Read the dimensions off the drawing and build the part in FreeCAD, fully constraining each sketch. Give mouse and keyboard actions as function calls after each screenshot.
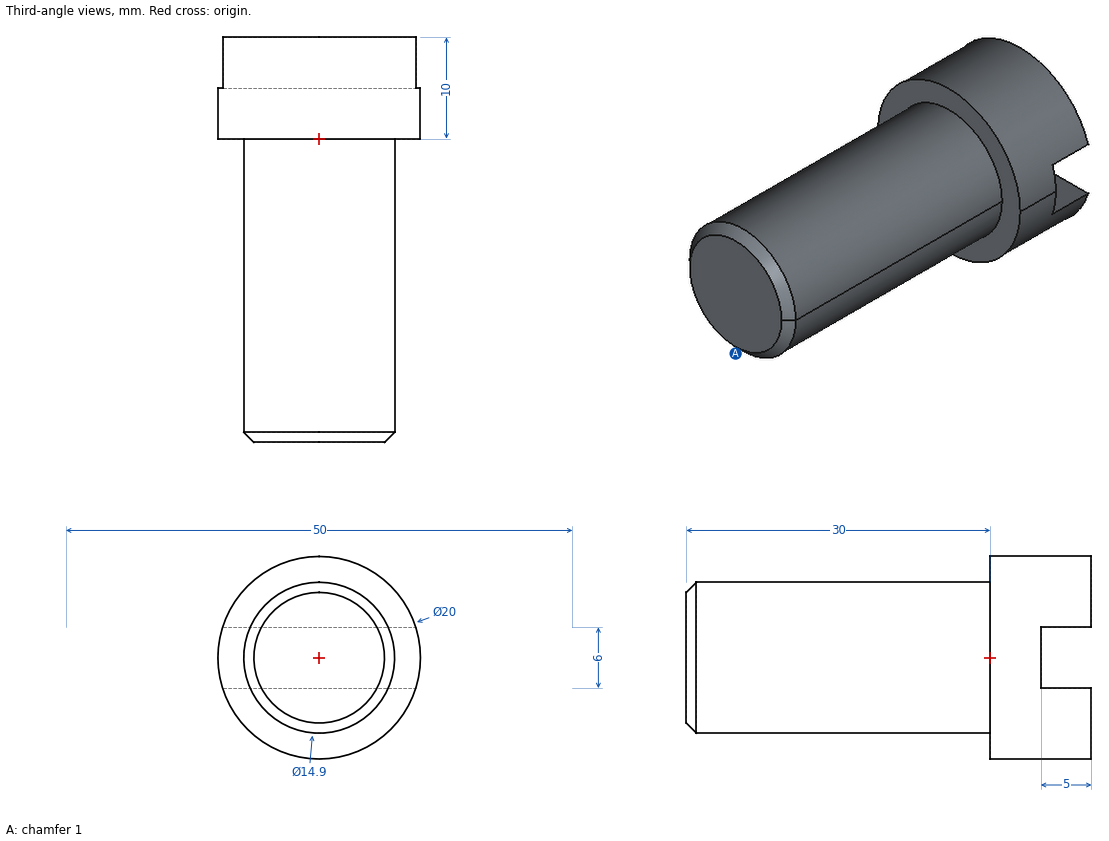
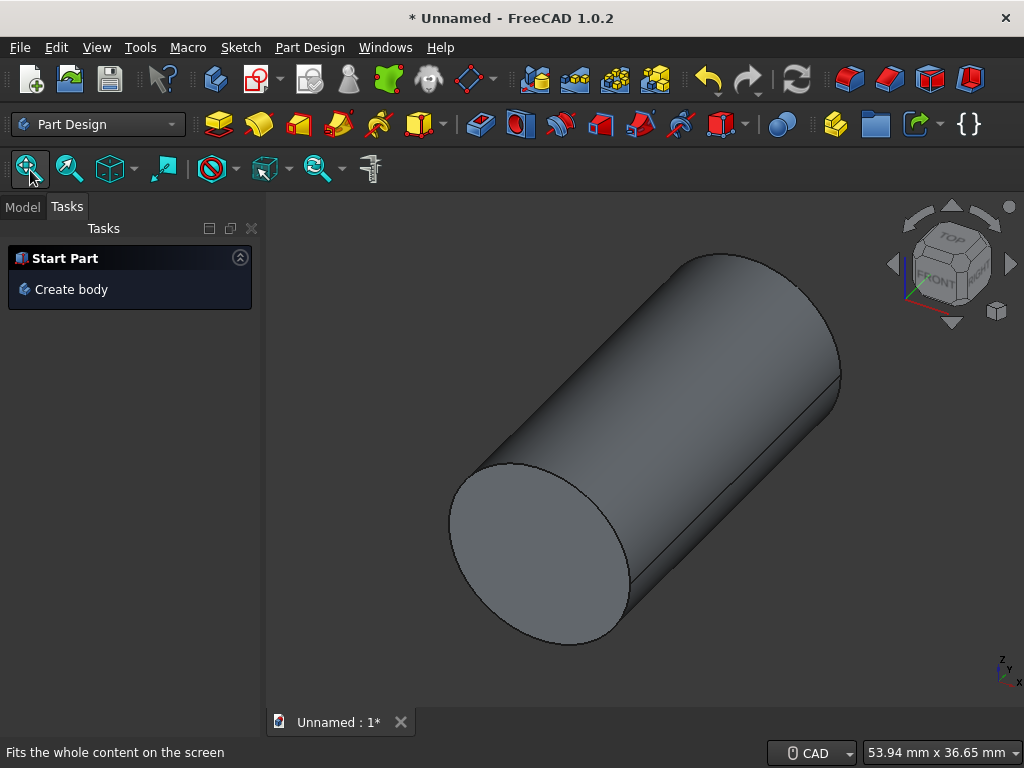
click(256, 80)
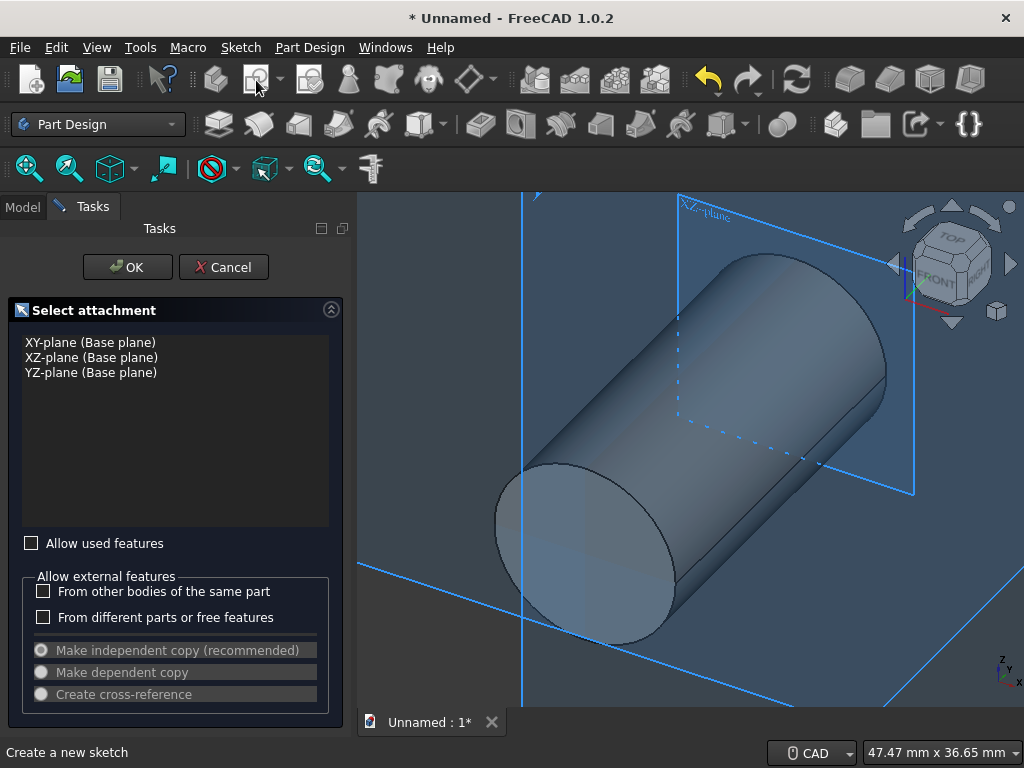
click(82, 358)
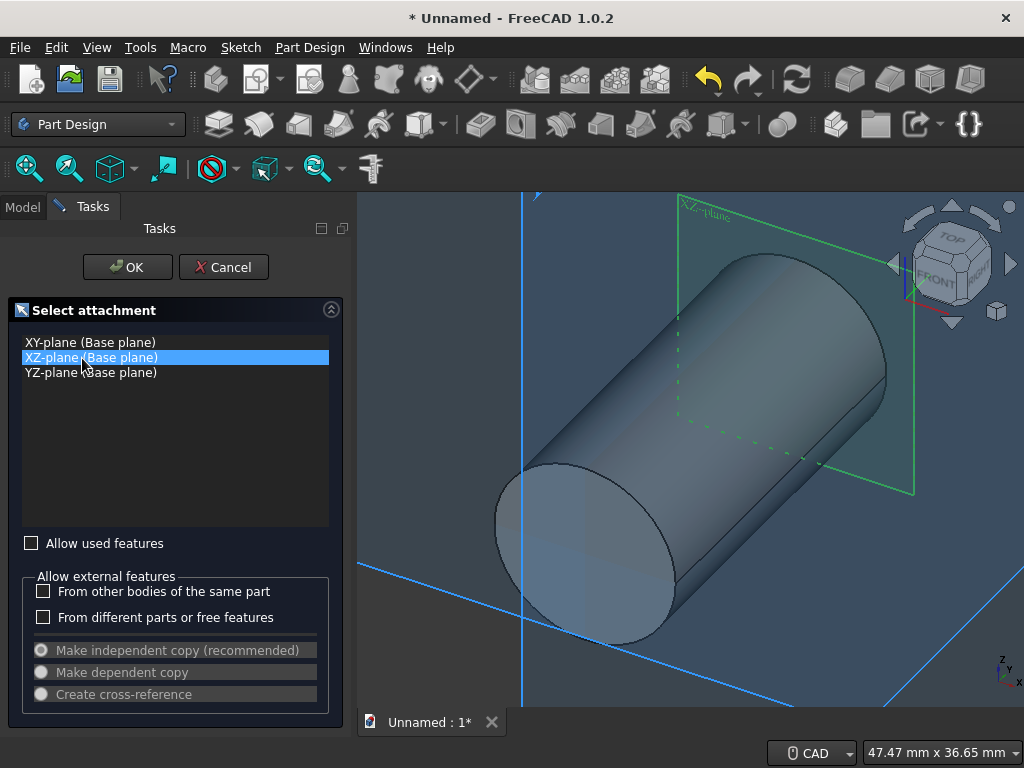
click(128, 267)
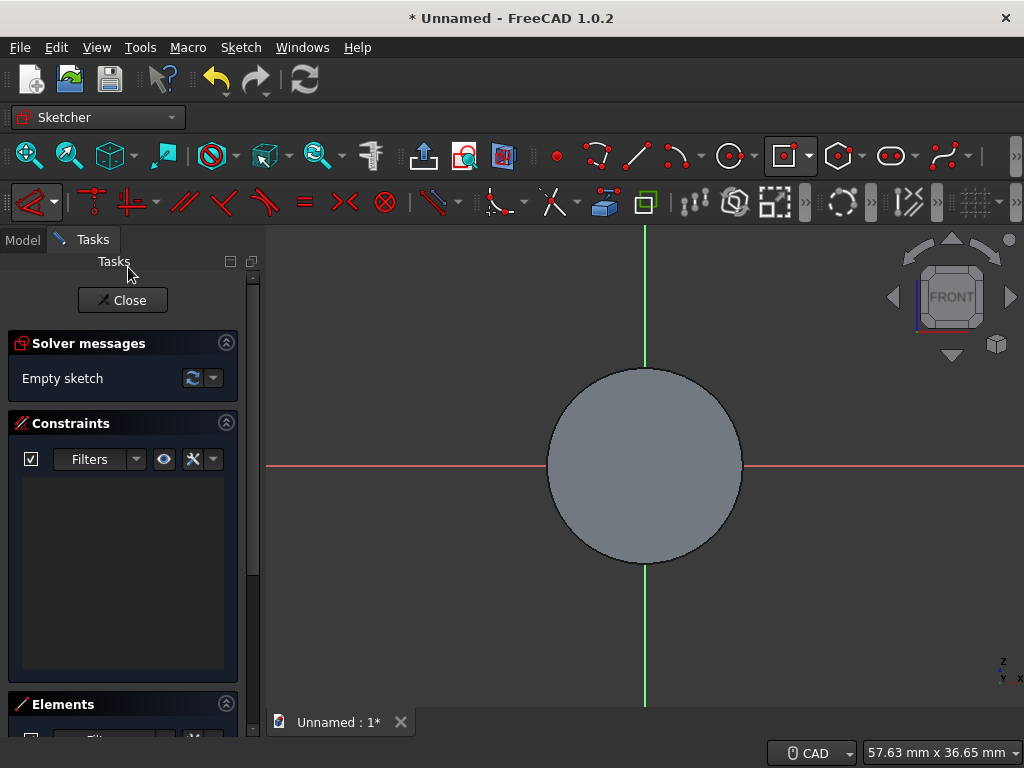
click(504, 156)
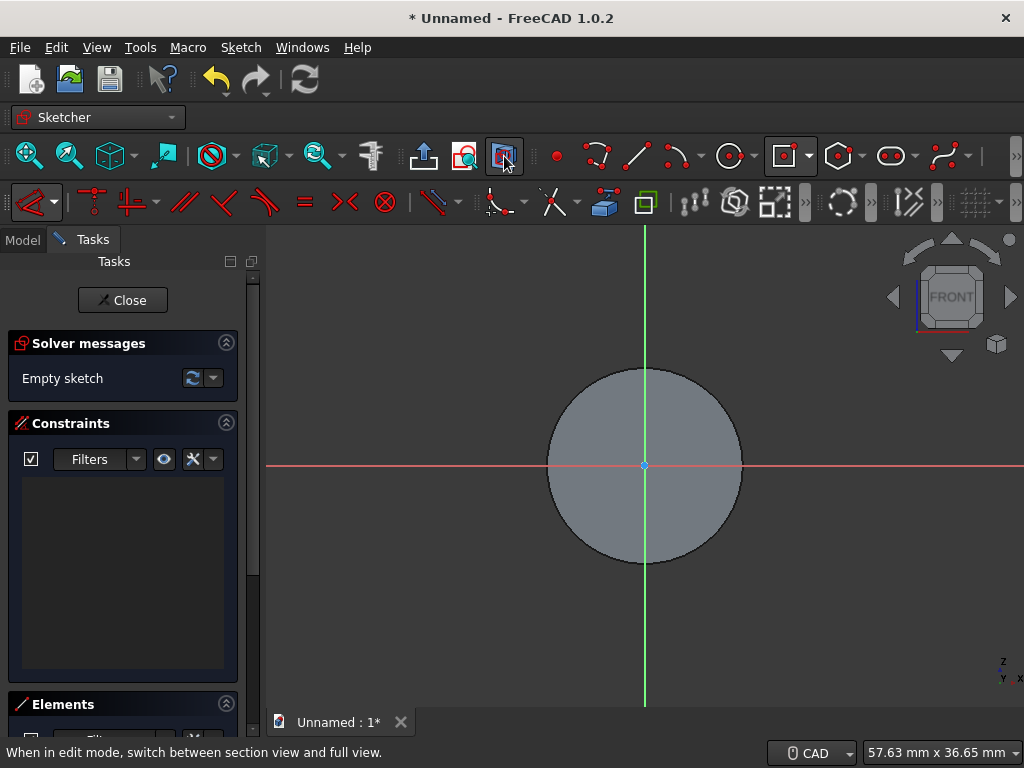
click(730, 156)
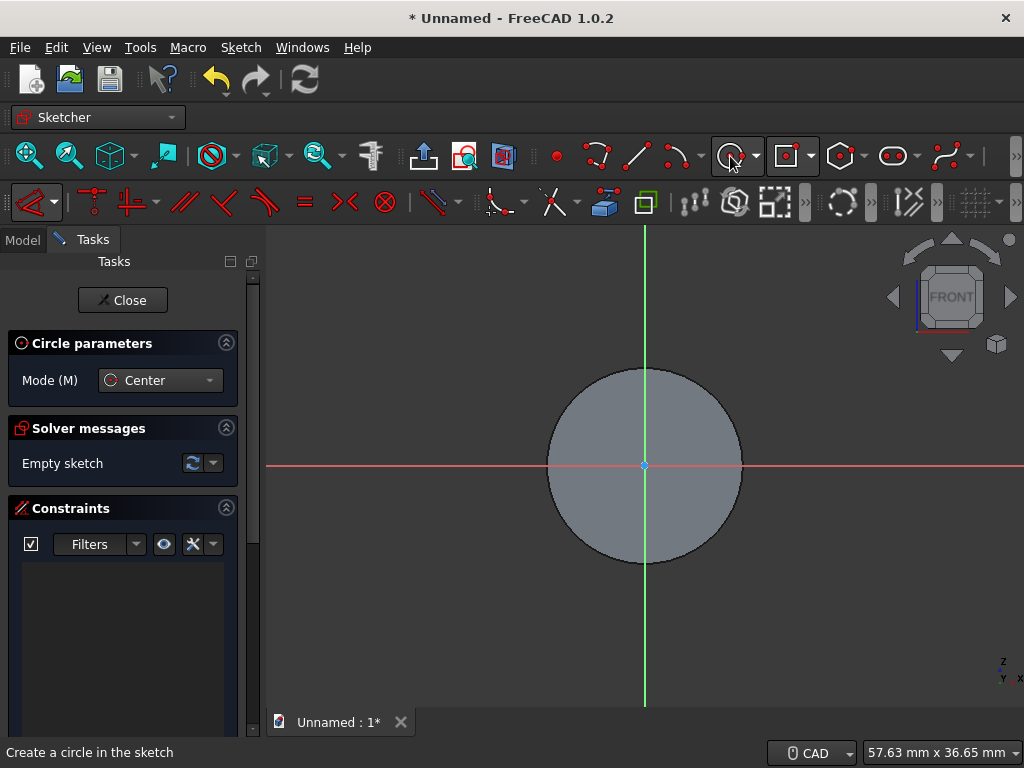
click(645, 466)
move(738, 373)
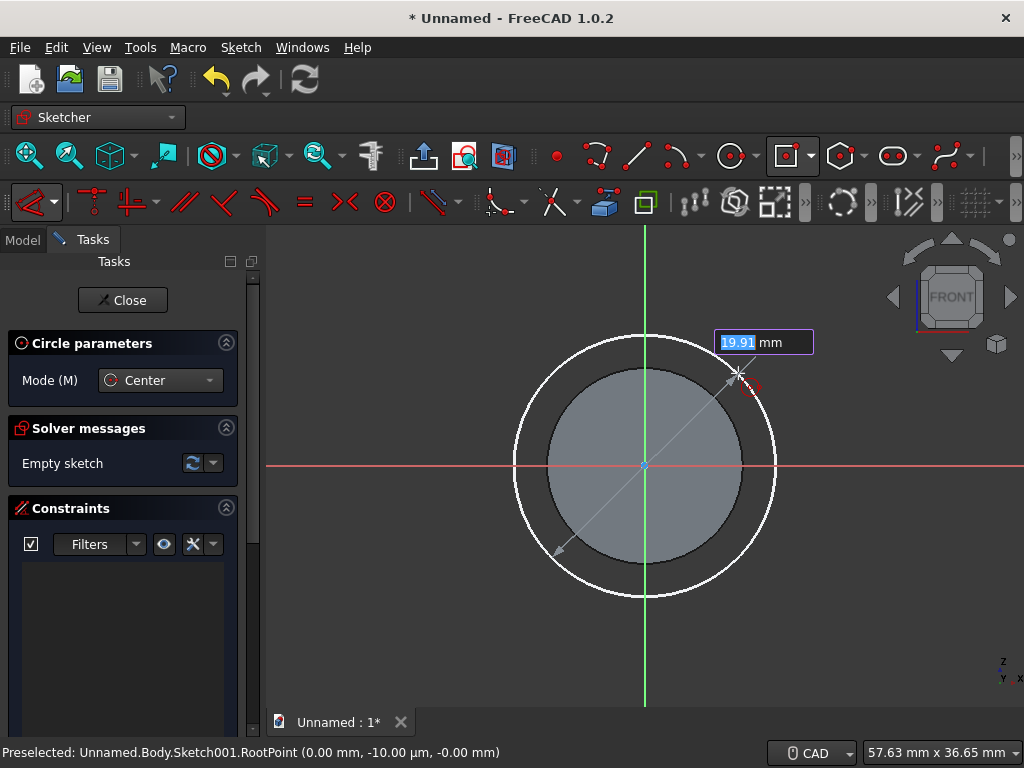
text(20)
key(Return)
key(Escape)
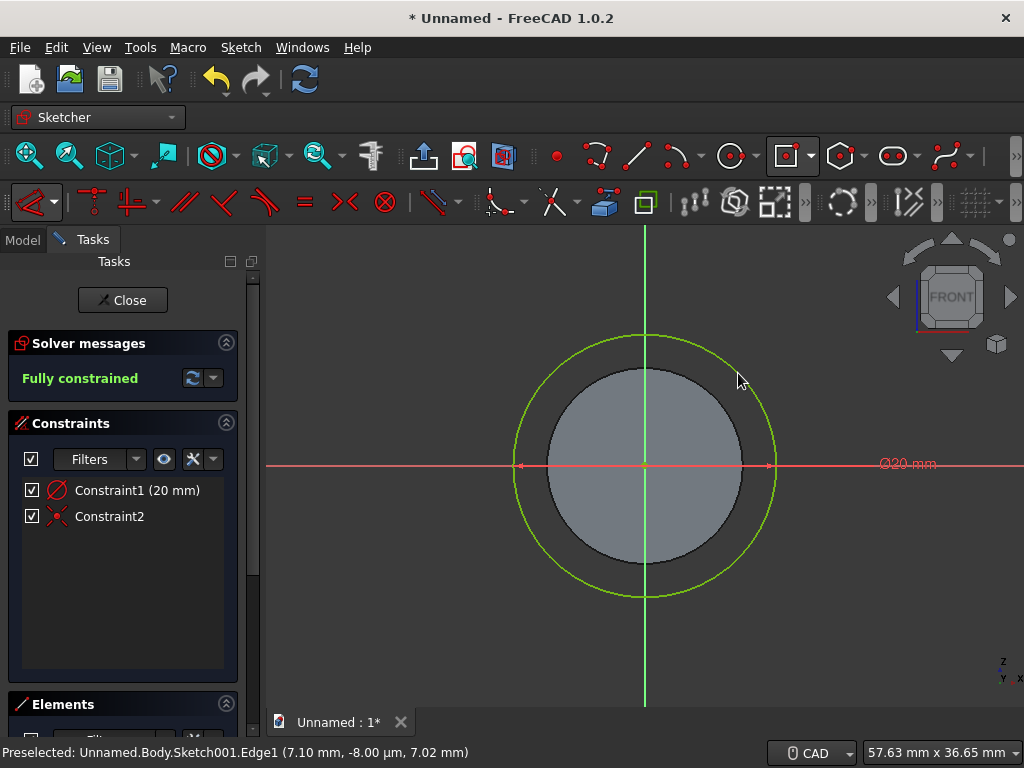
click(123, 300)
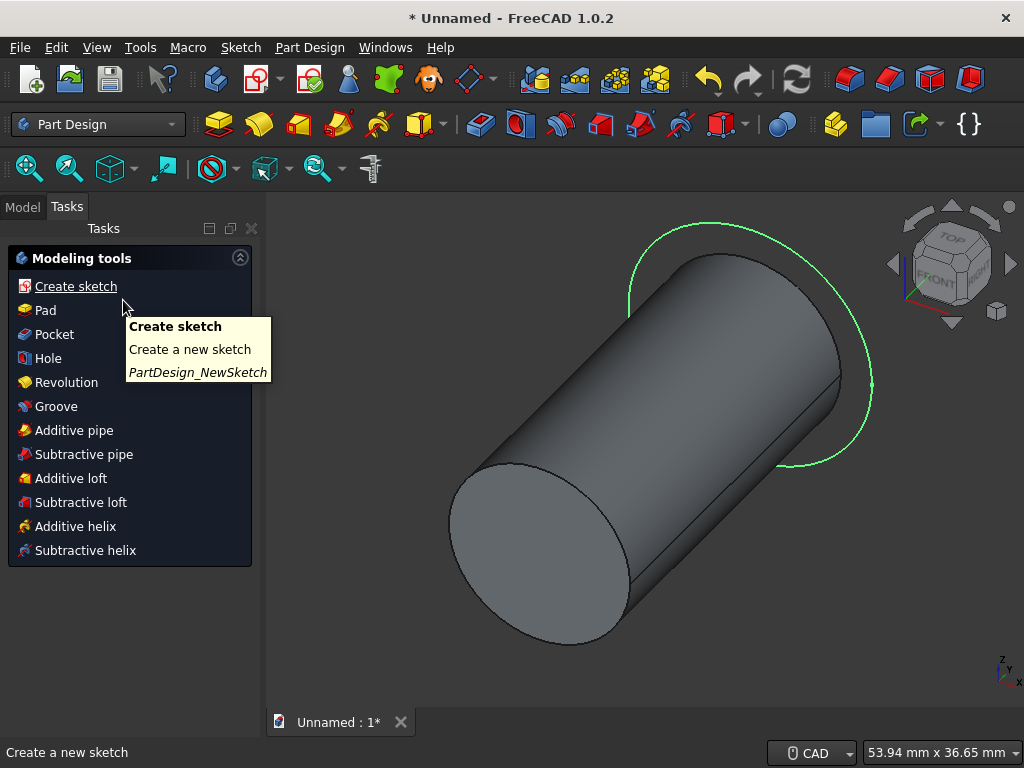
click(220, 124)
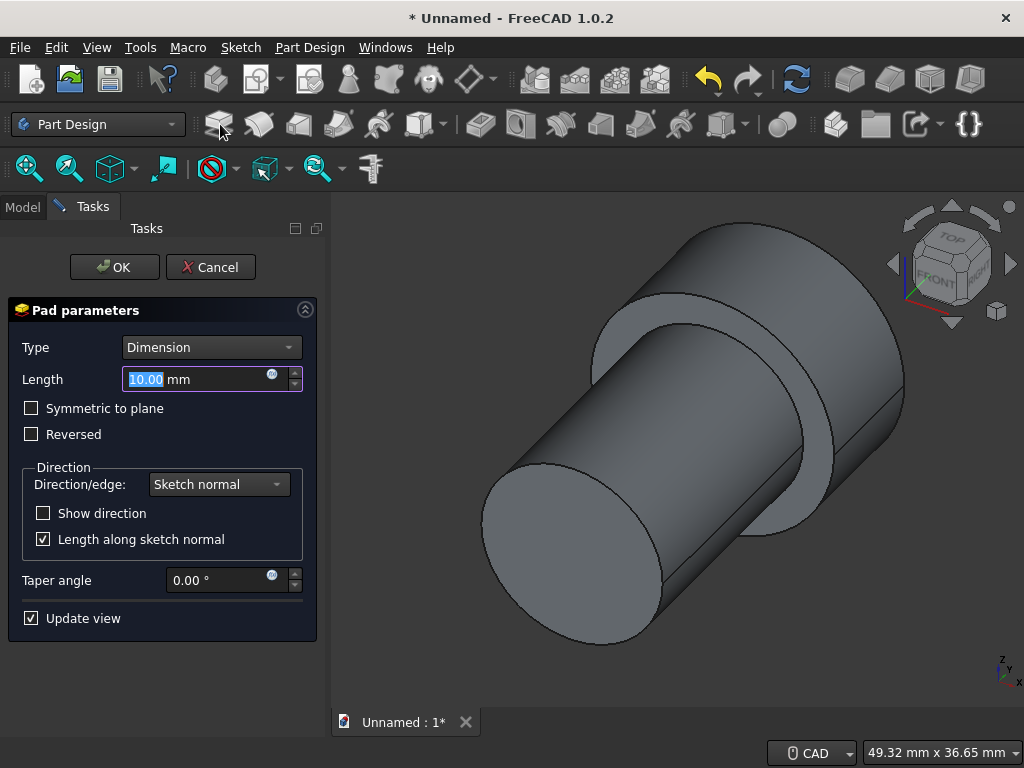
text(10)
key(Tab)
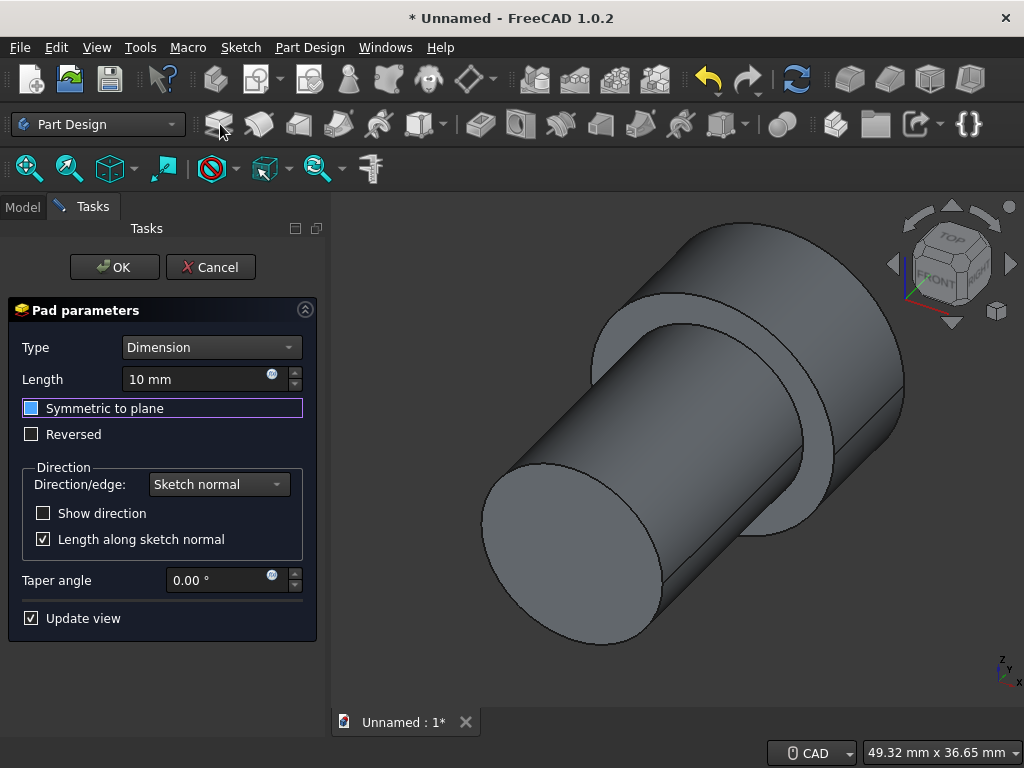
click(30, 434)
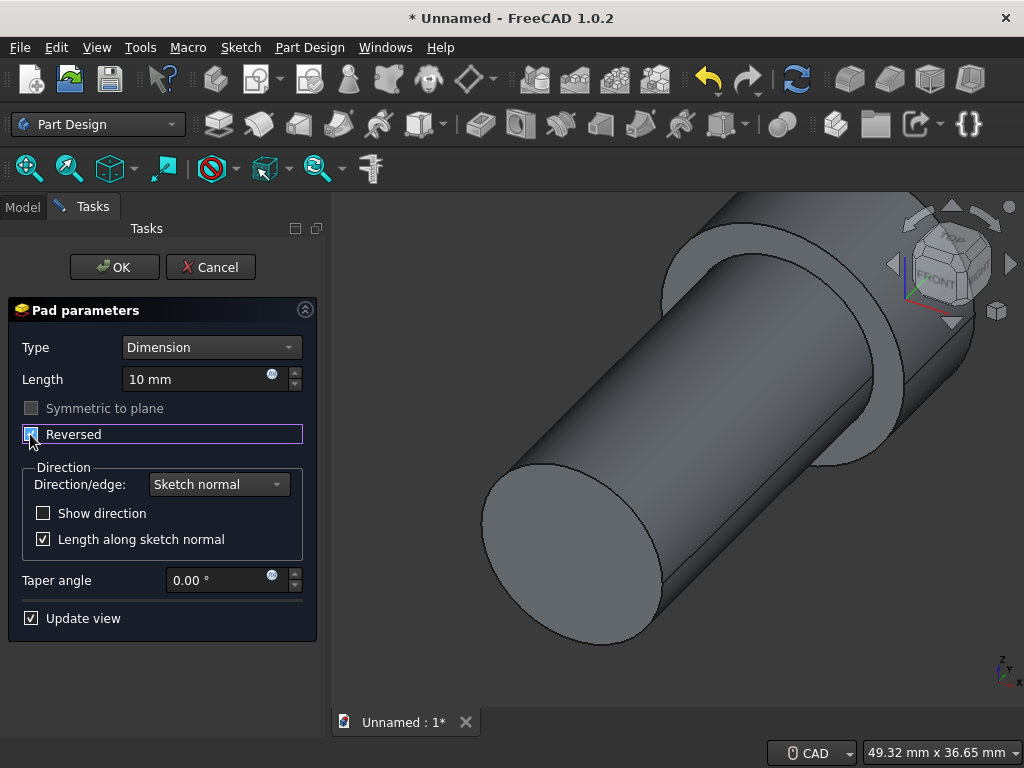
click(115, 267)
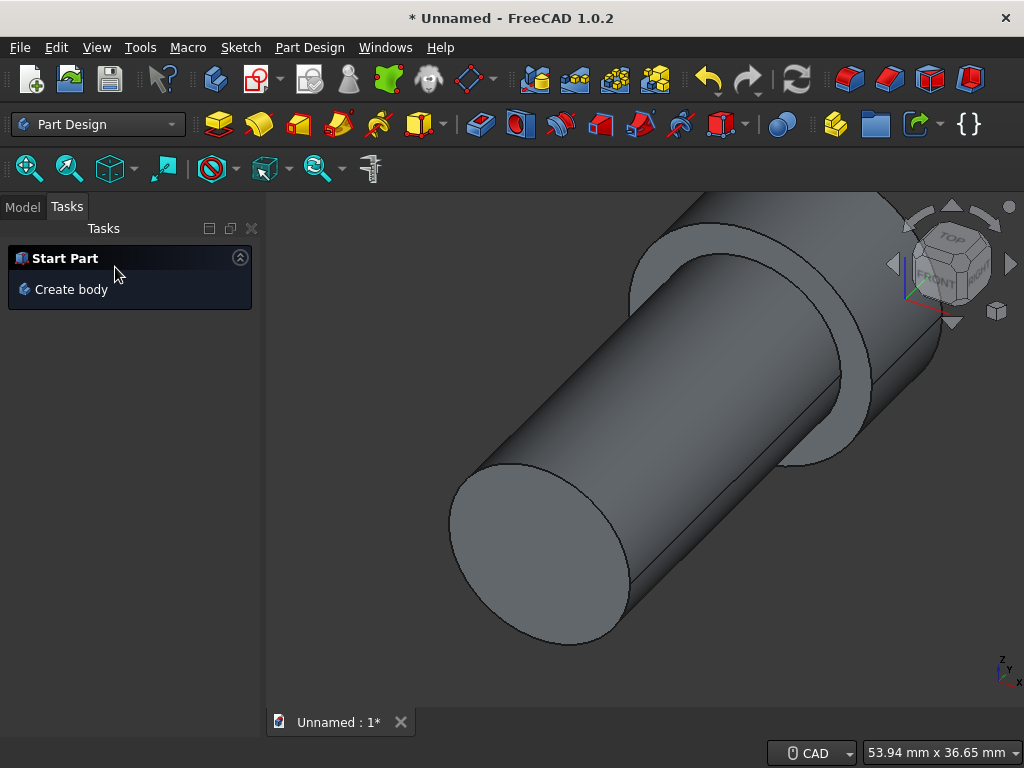
click(30, 170)